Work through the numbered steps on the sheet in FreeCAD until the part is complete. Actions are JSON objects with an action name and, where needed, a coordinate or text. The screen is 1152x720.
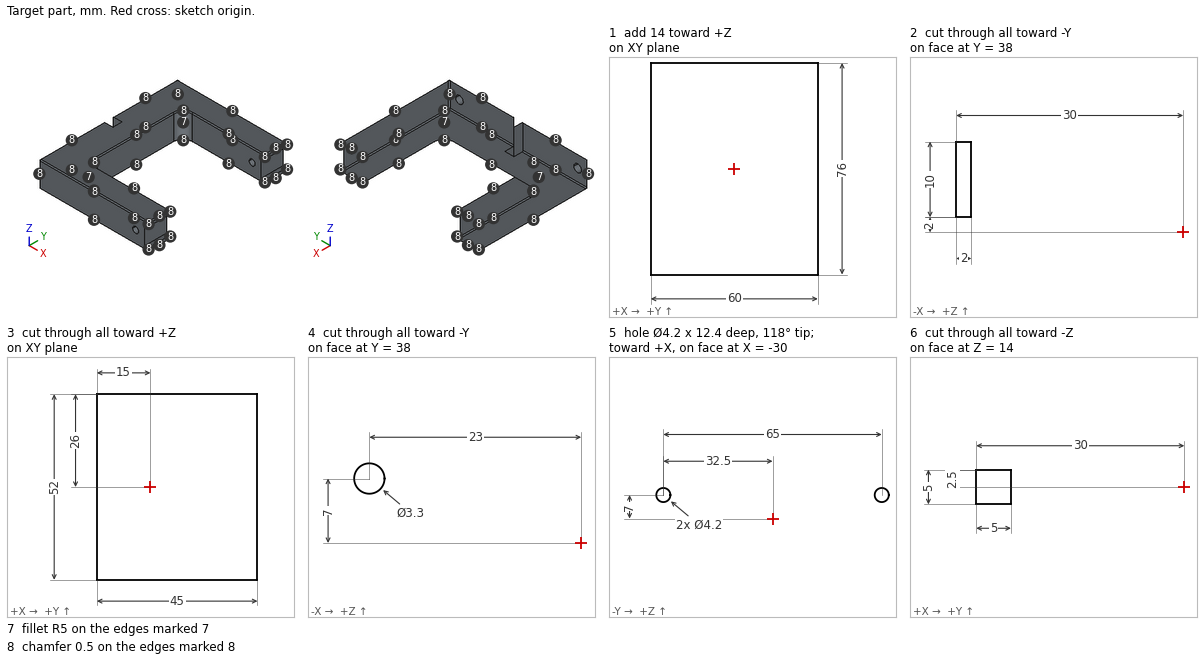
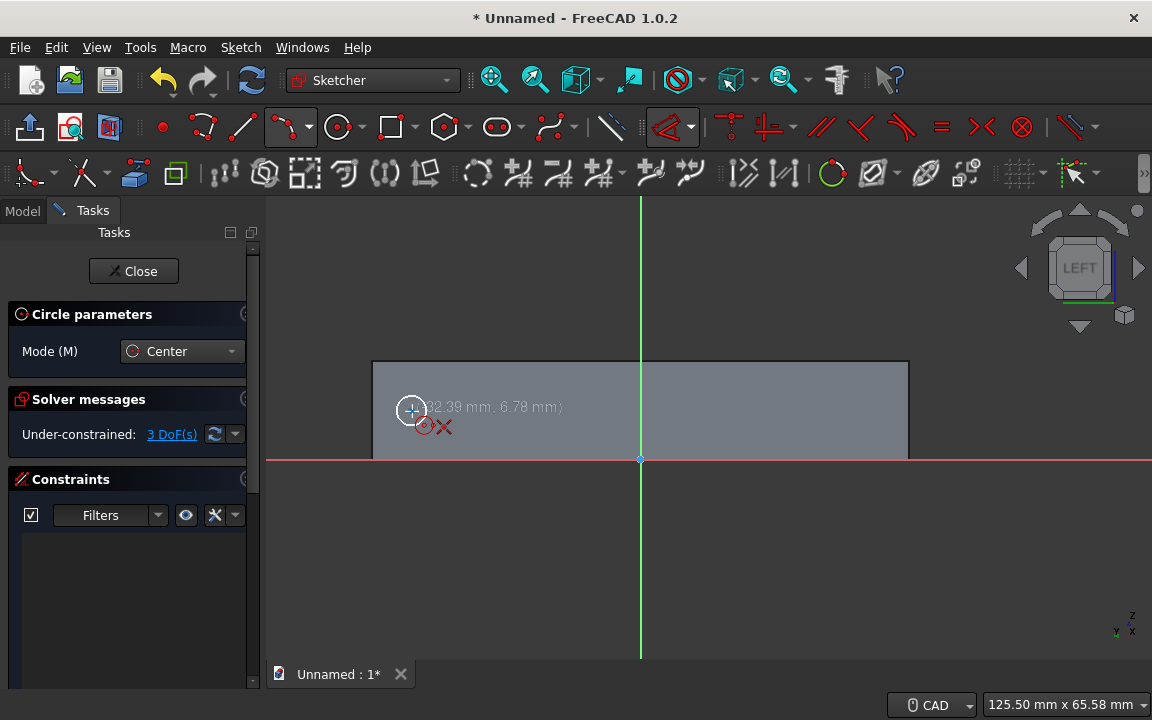
{"action": "scroll", "coordinate": [870, 410], "scroll_direction": "up", "scroll_amount": 3}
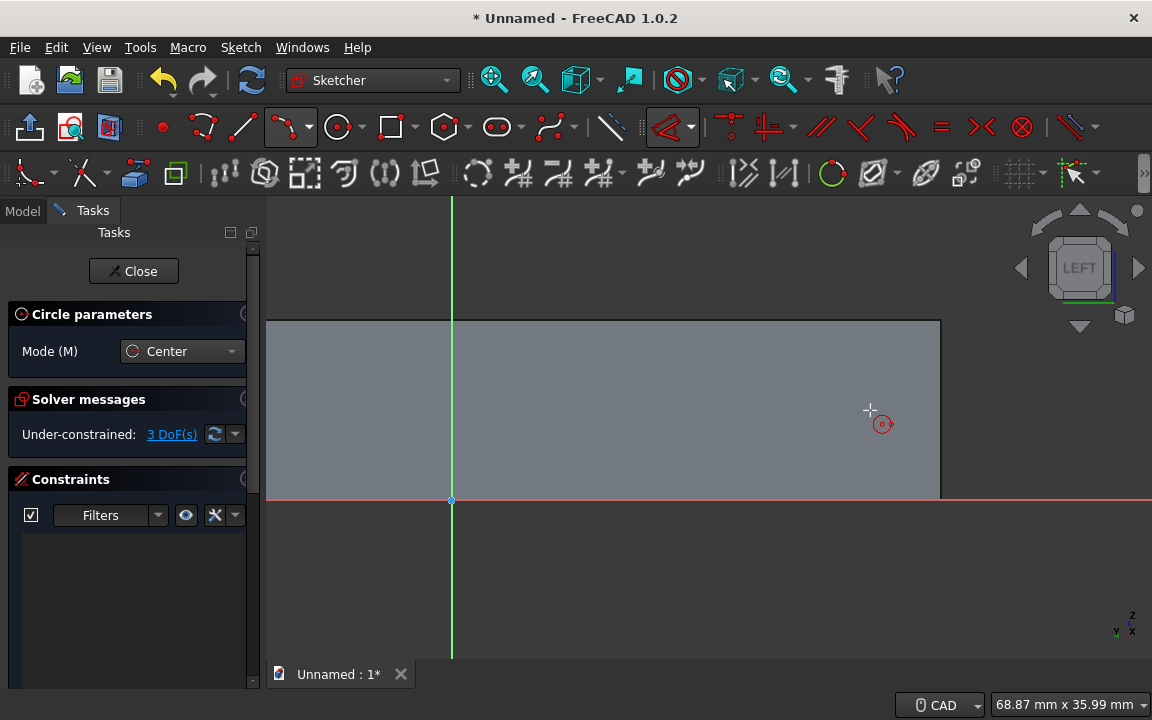
{"action": "left_click", "coordinate": [870, 410]}
{"action": "left_click", "coordinate": [889, 391]}
{"action": "key", "text": "Escape"}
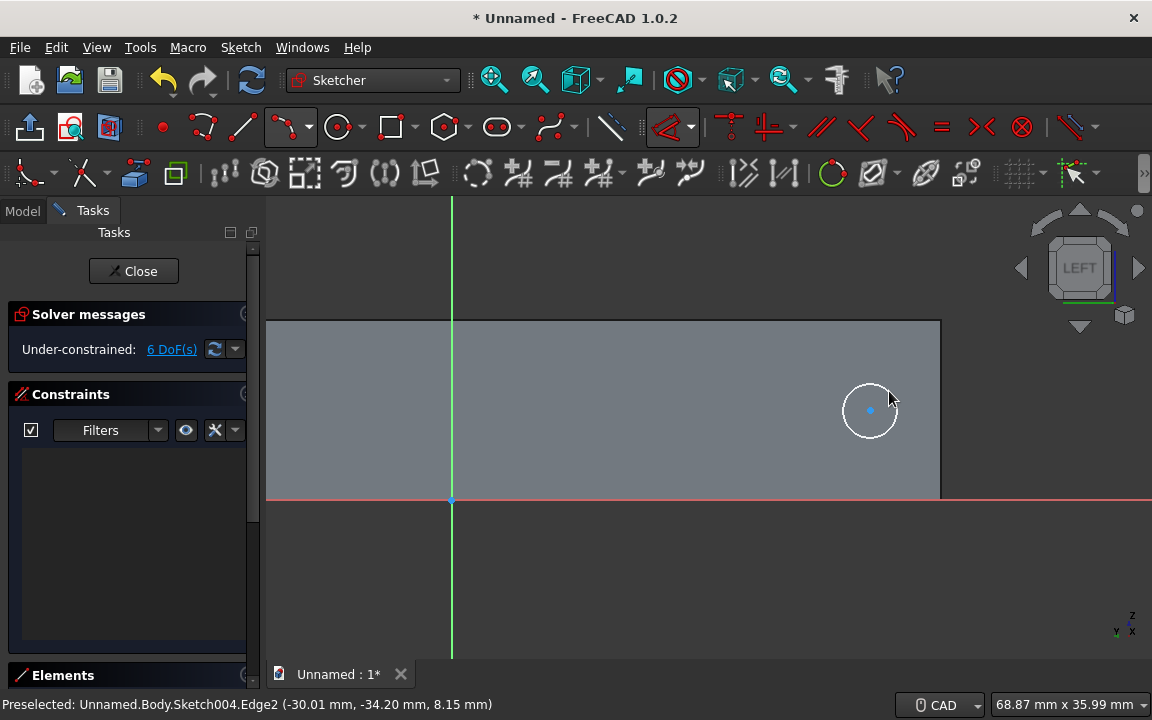
{"action": "scroll", "coordinate": [870, 410], "scroll_direction": "down", "scroll_amount": 3}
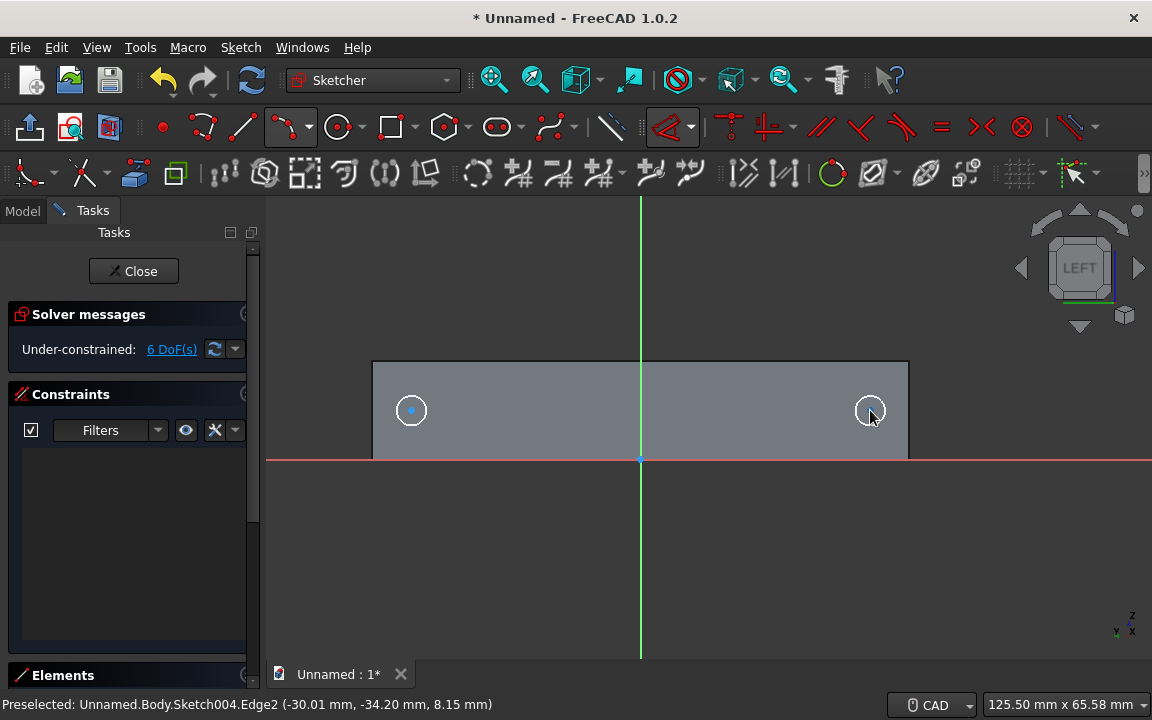
{"action": "left_click", "coordinate": [422, 400]}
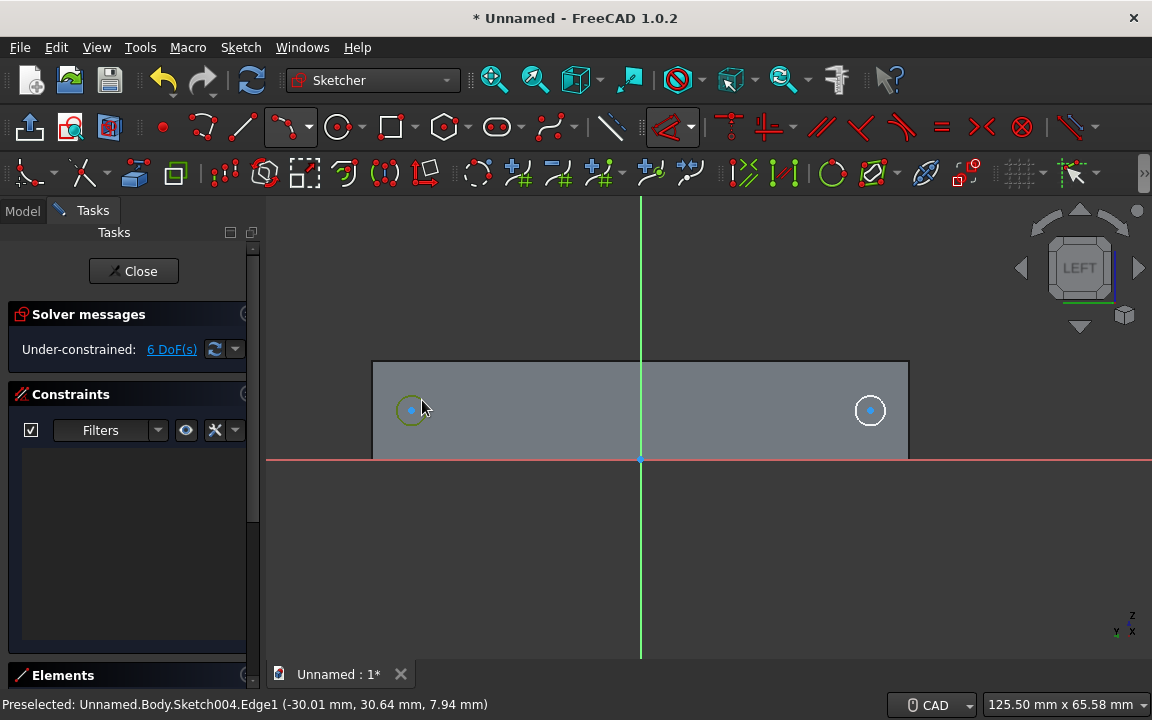
{"action": "left_click", "coordinate": [881, 400]}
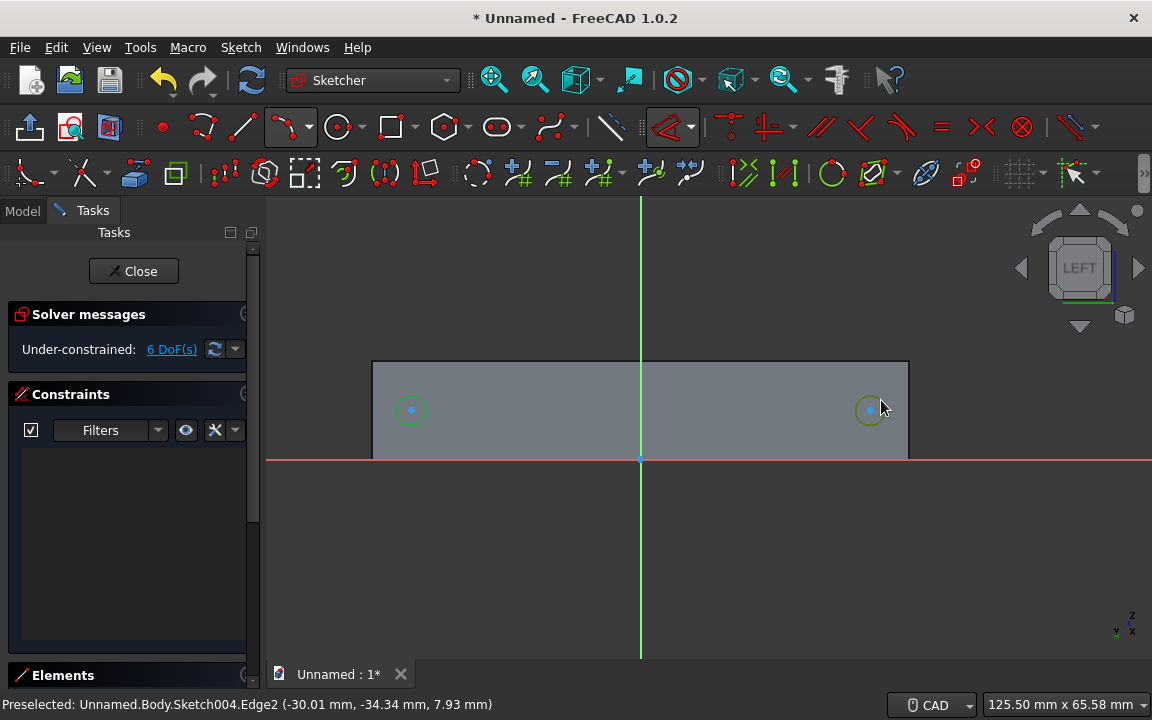
{"action": "left_click", "coordinate": [942, 128]}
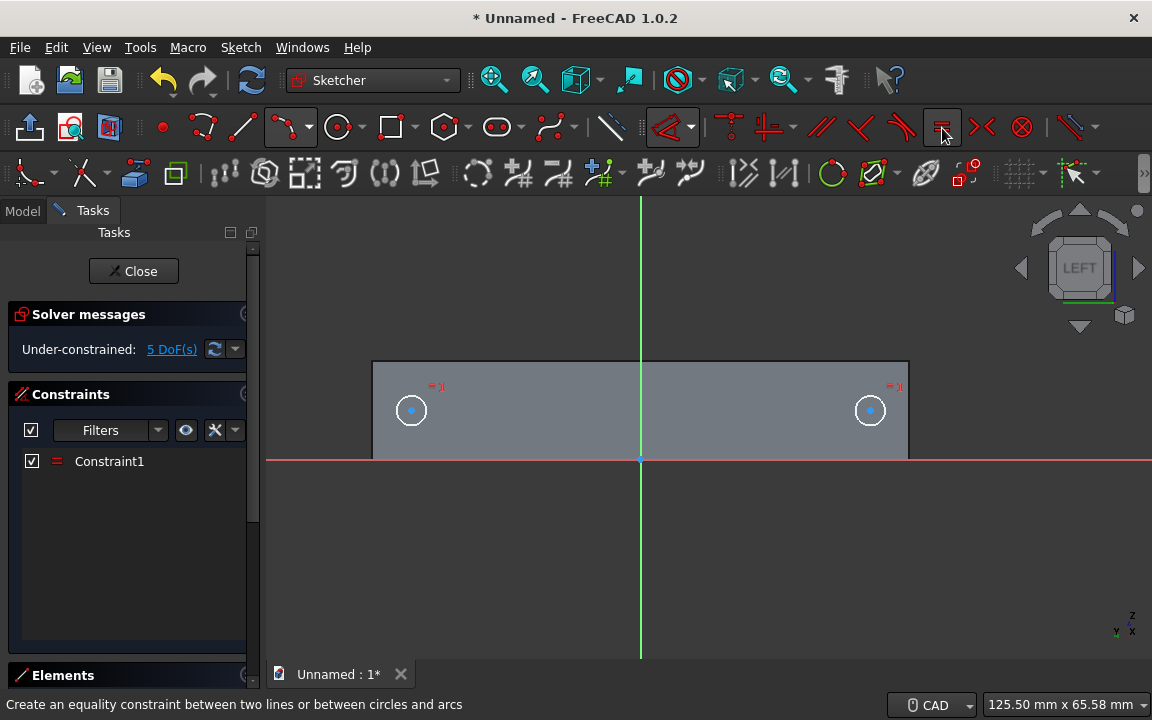
{"action": "left_click", "coordinate": [412, 411]}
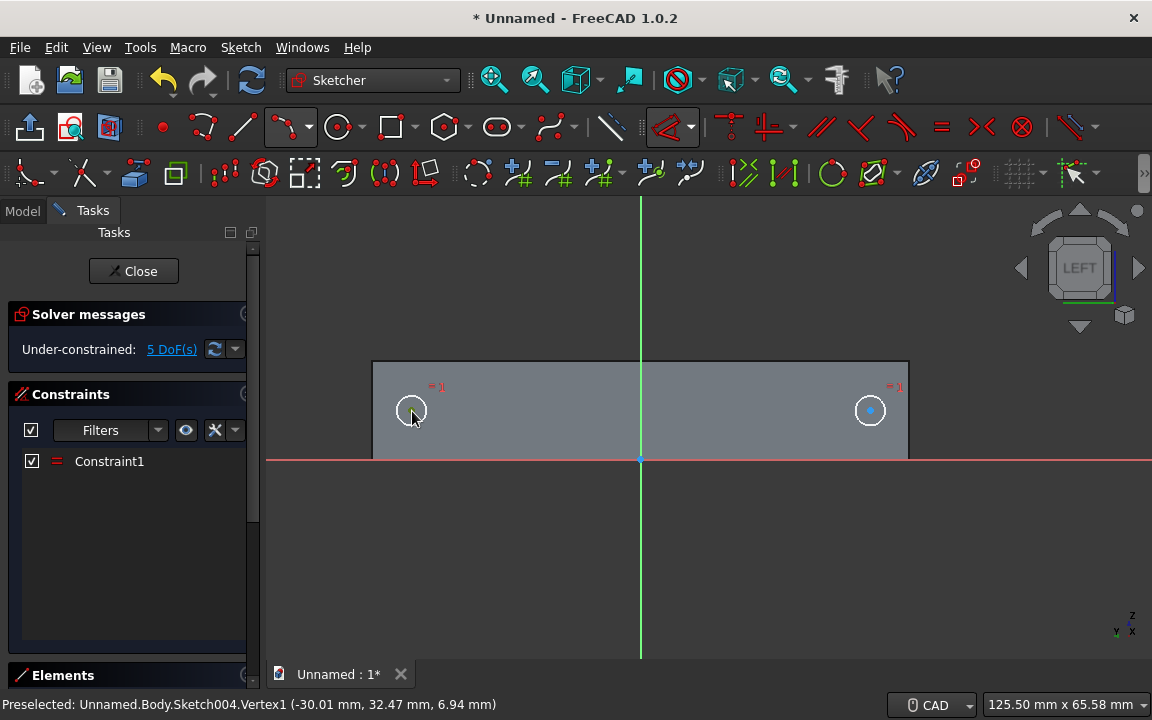
{"action": "left_click", "coordinate": [870, 411]}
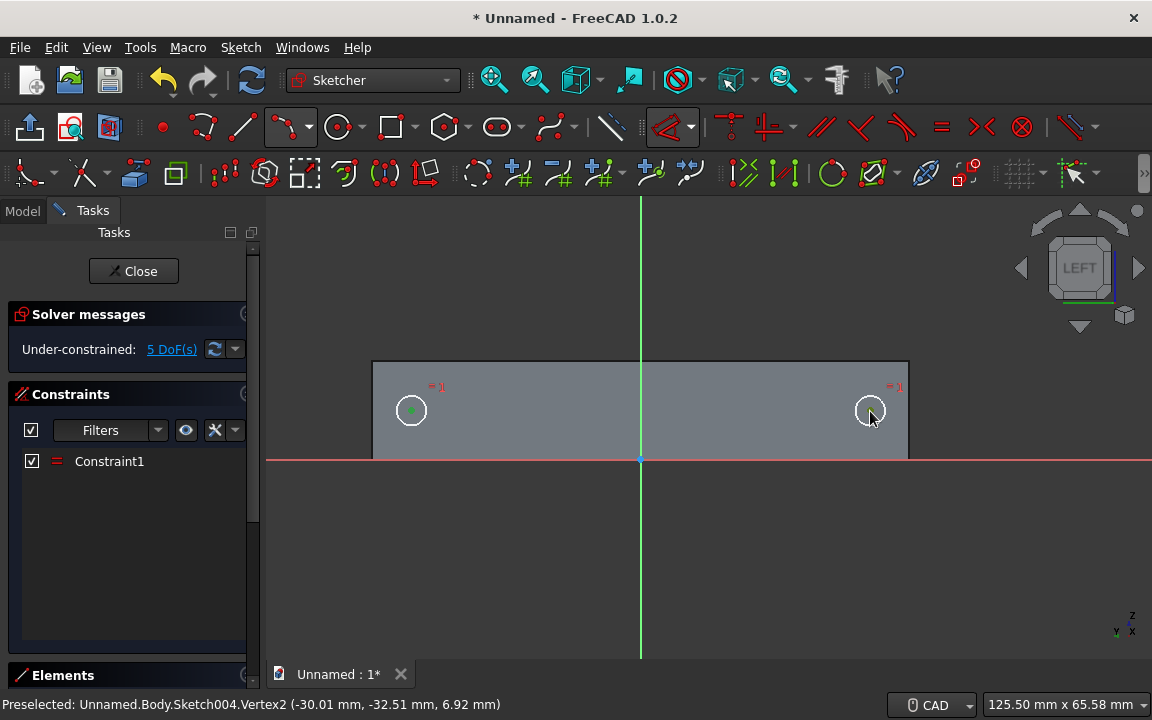
{"action": "key", "text": "h"}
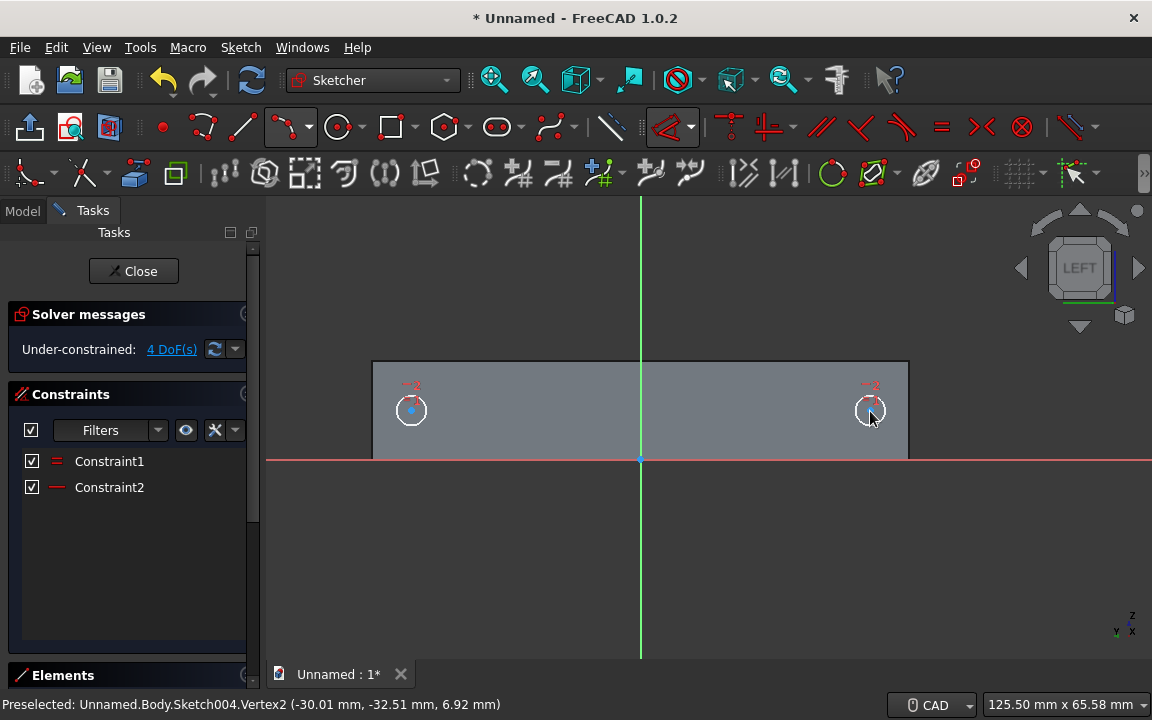
{"action": "scroll", "coordinate": [422, 400], "scroll_direction": "up", "scroll_amount": 2}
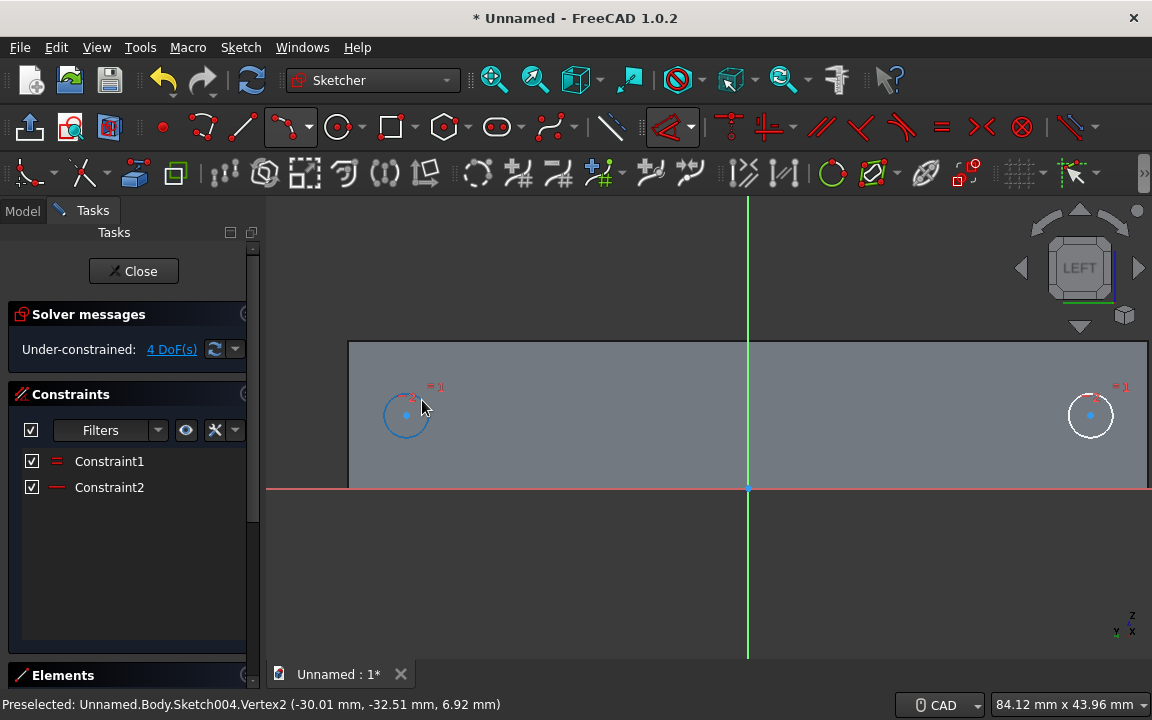
{"action": "left_click", "coordinate": [422, 400]}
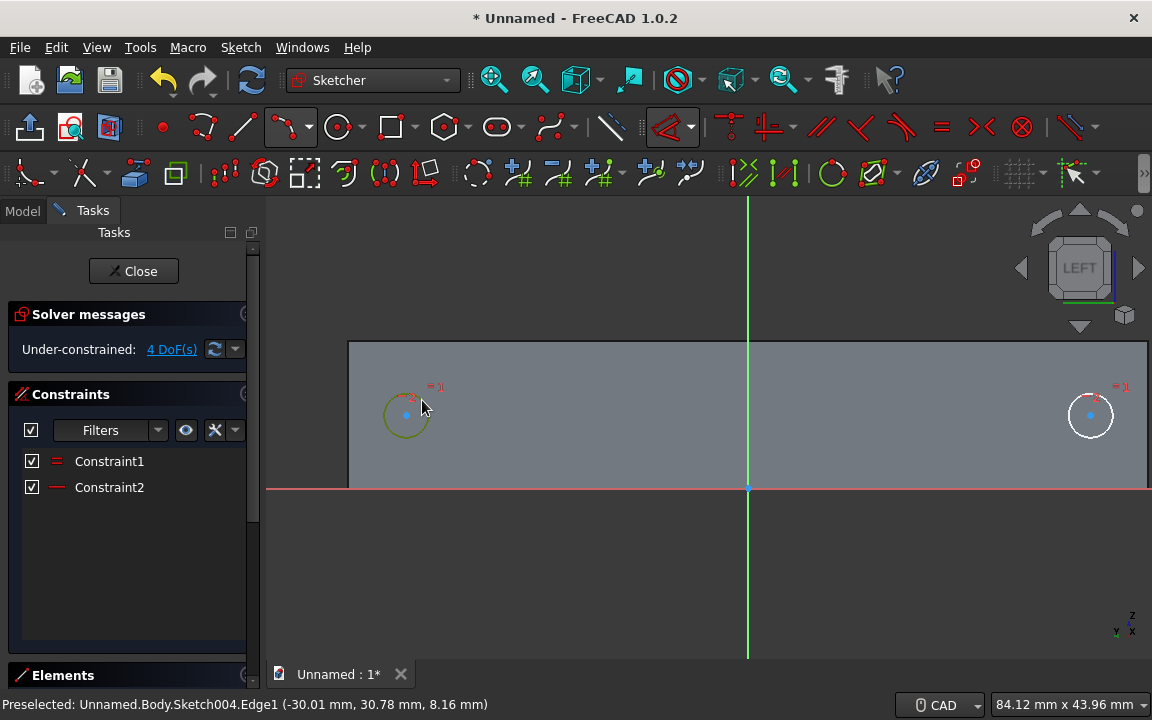
{"action": "left_click", "coordinate": [694, 128]}